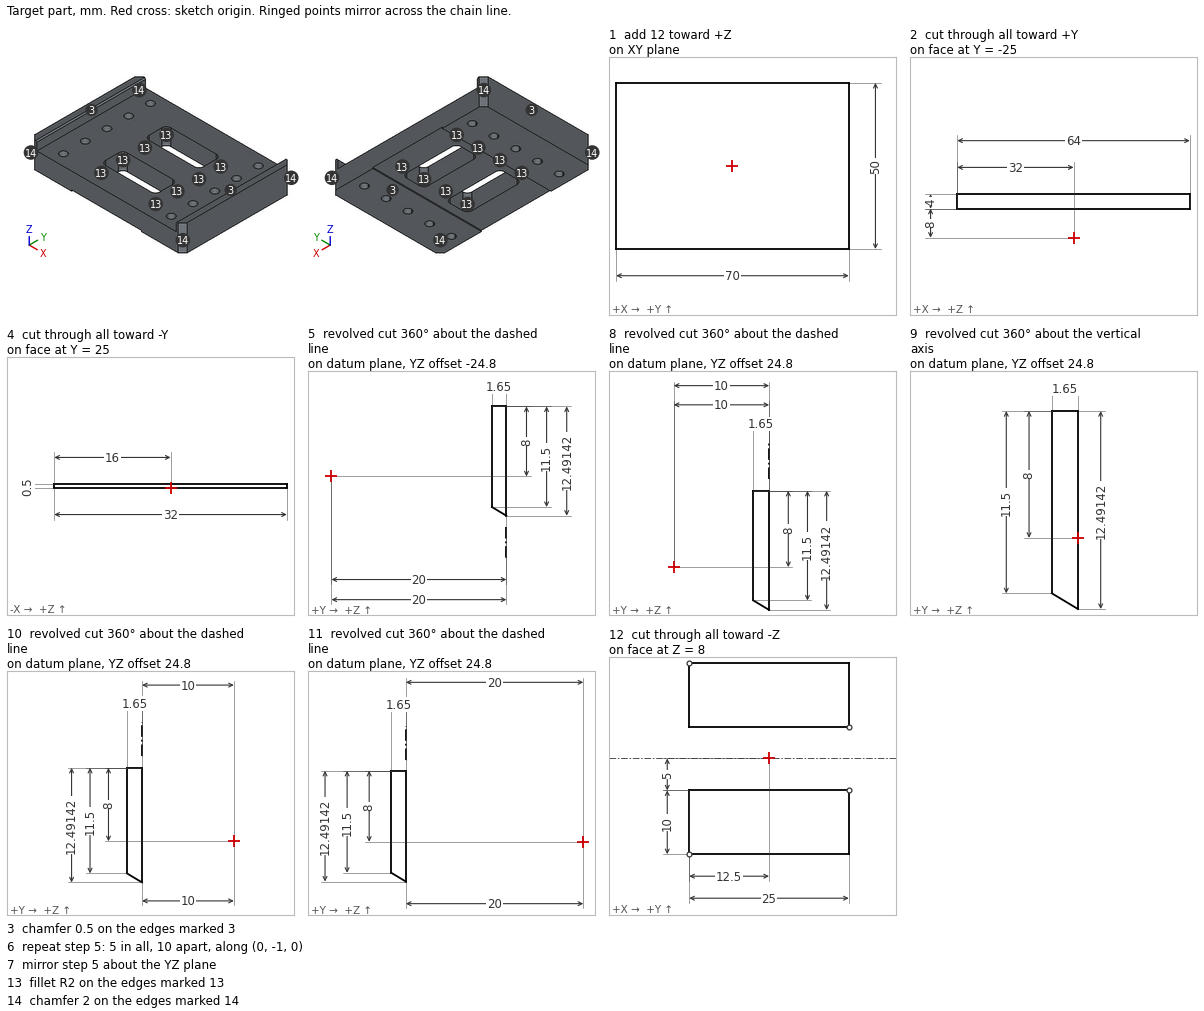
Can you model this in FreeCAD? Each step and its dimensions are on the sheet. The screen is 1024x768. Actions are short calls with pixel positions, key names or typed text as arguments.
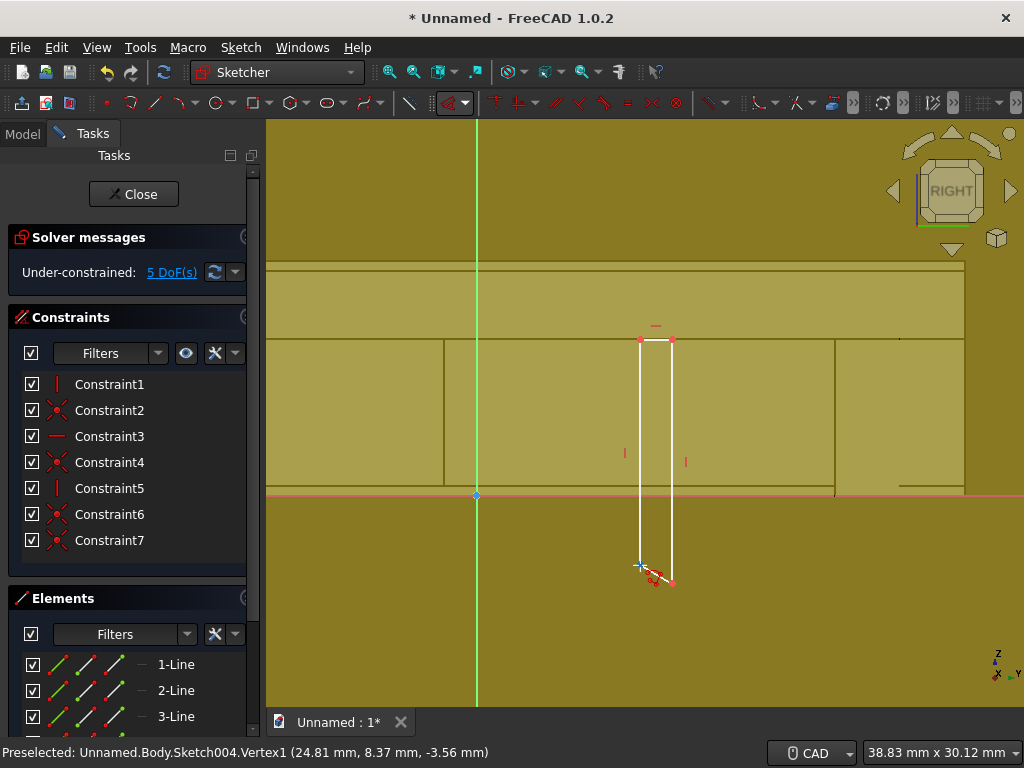
key(g)
key(l)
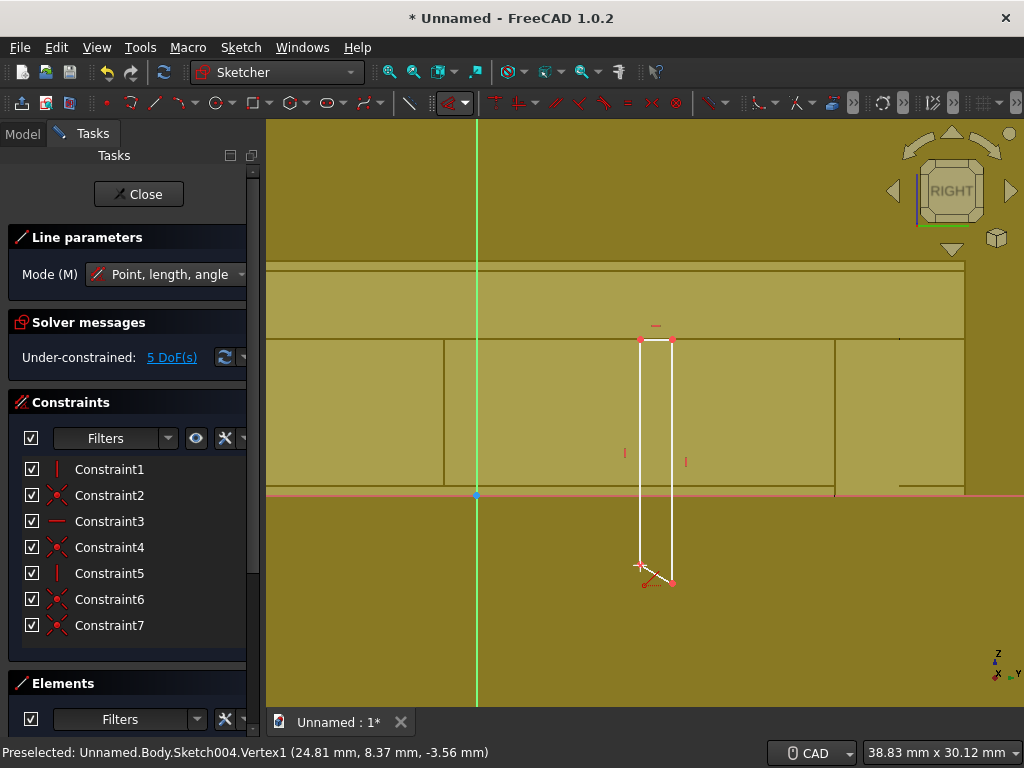
click(672, 315)
click(672, 242)
key(Escape)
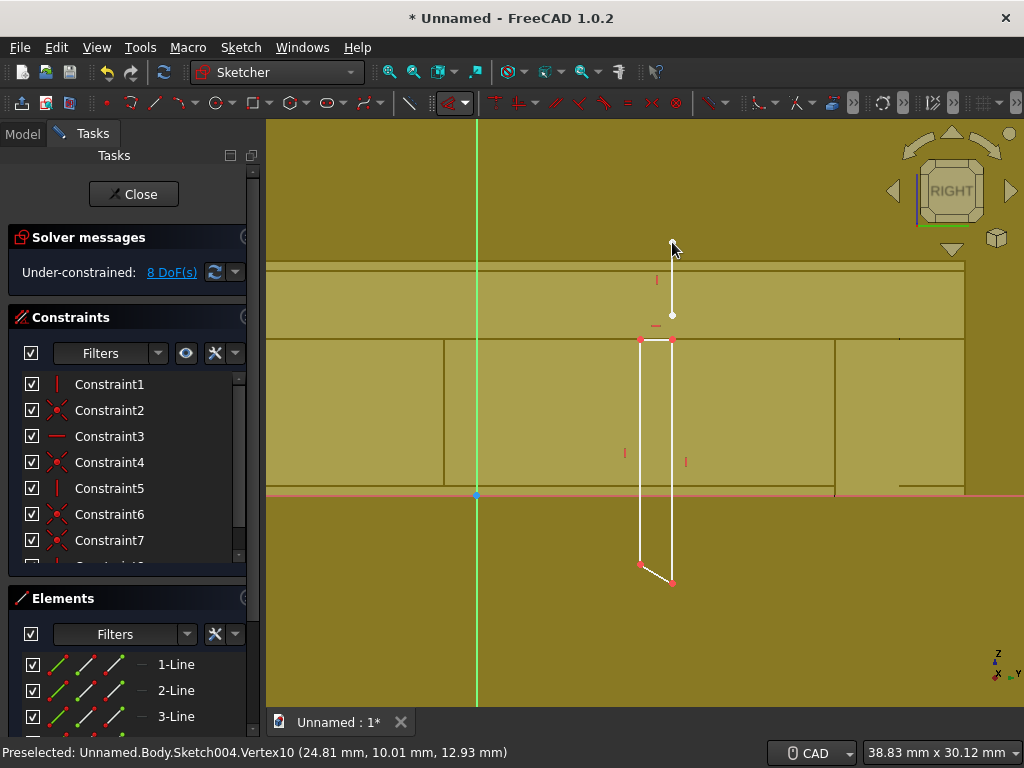
click(672, 294)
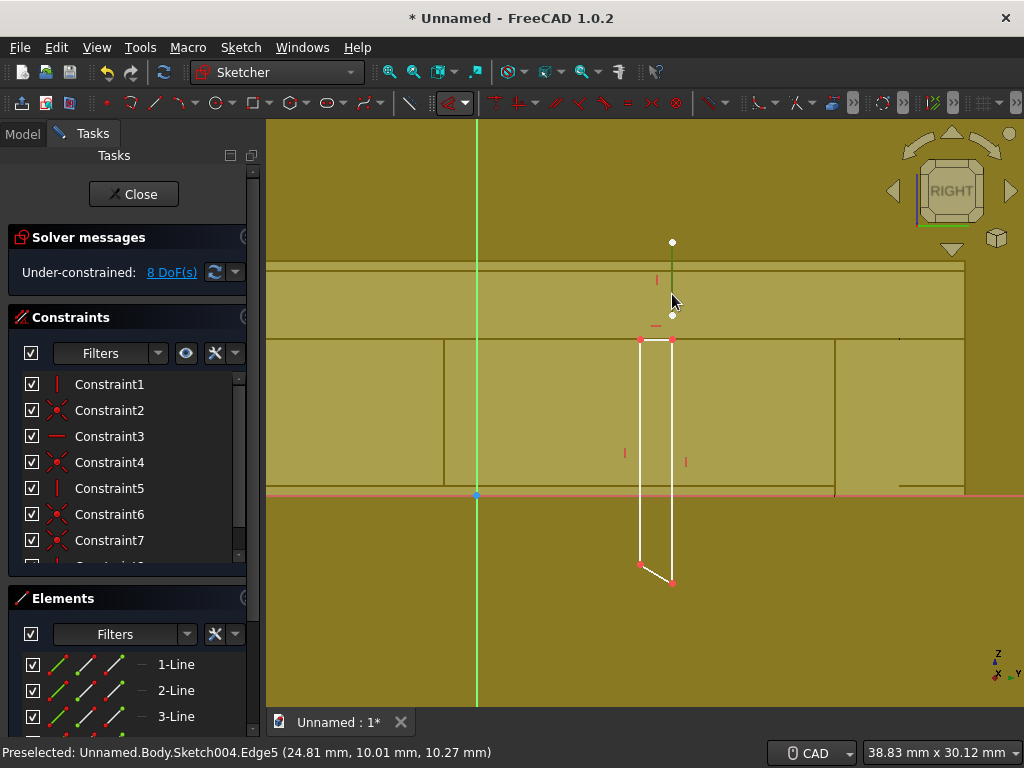
key(g)
key(n)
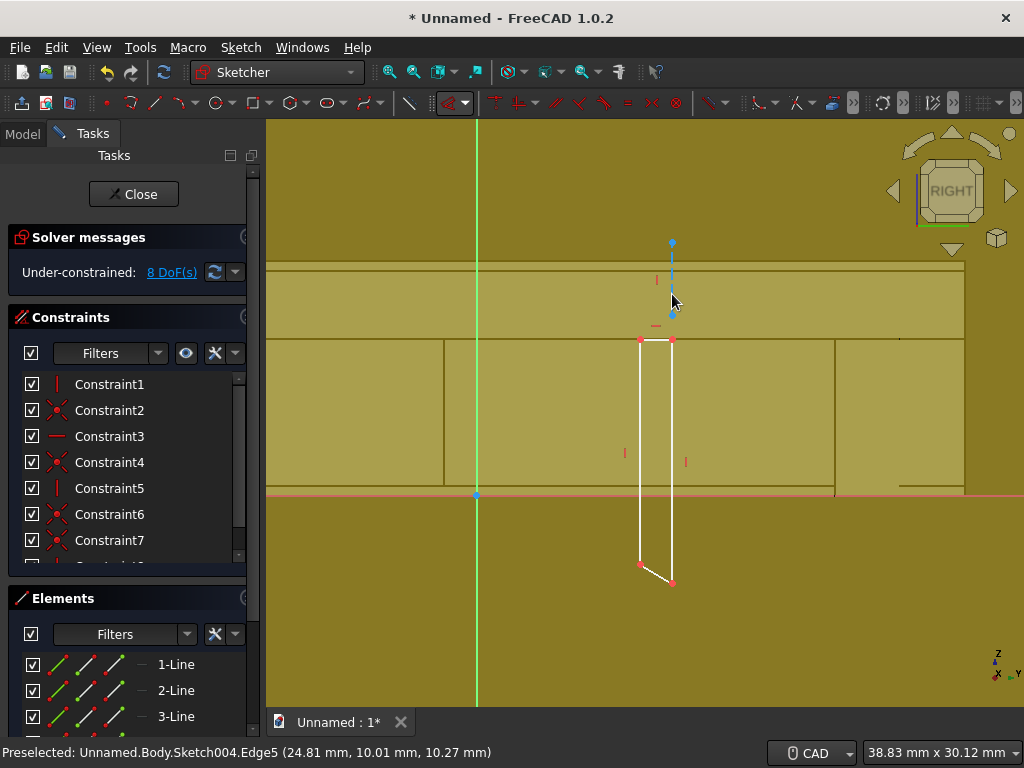
click(640, 340)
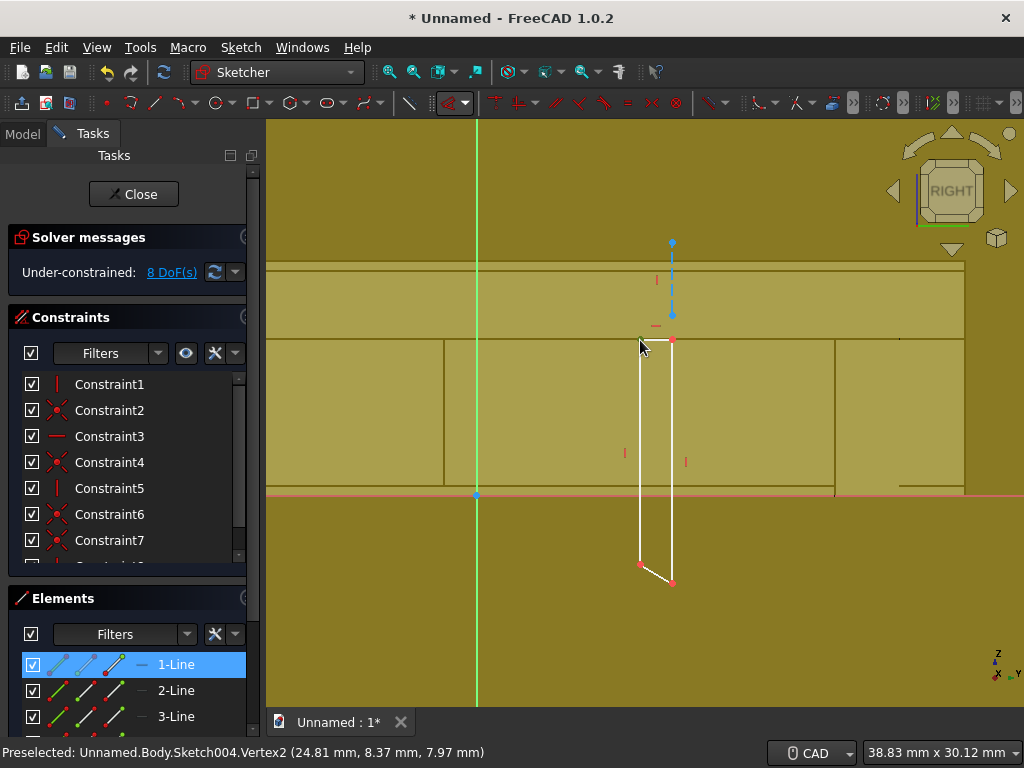
key(i)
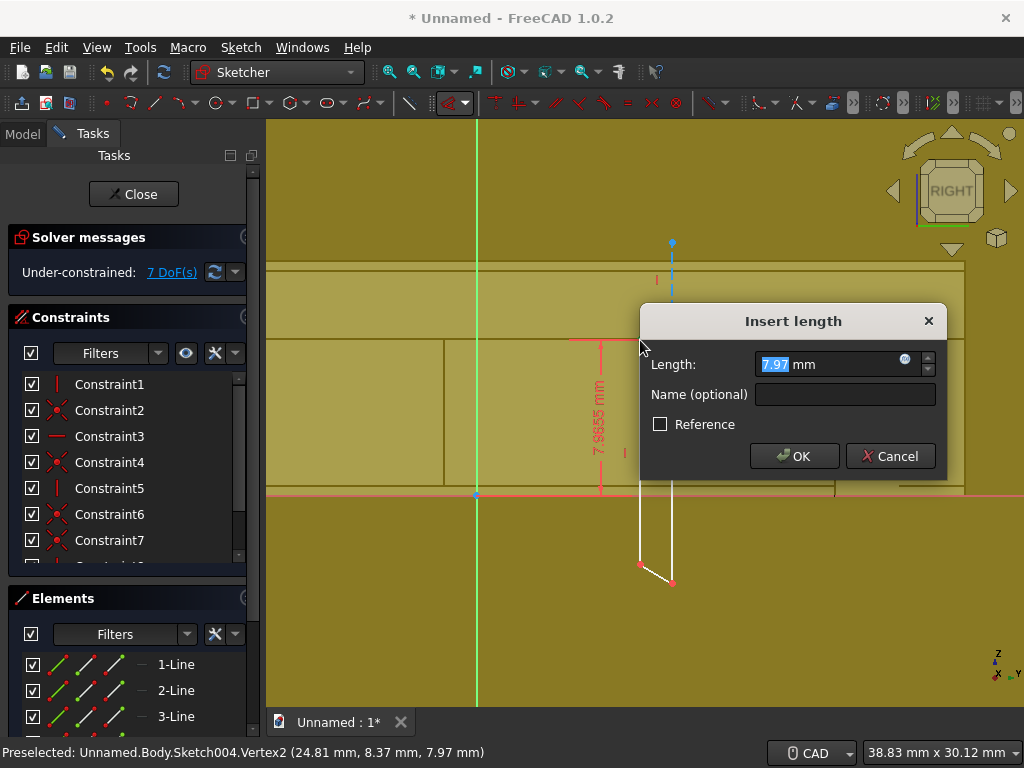
text(8)
key(Return)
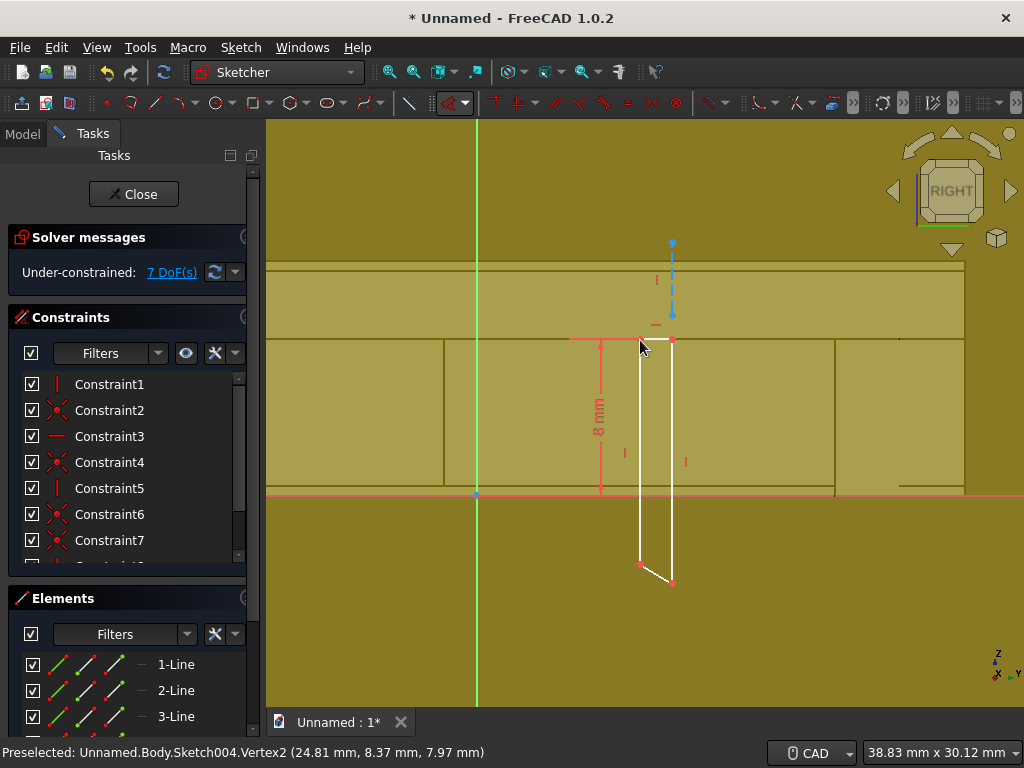
click(672, 339)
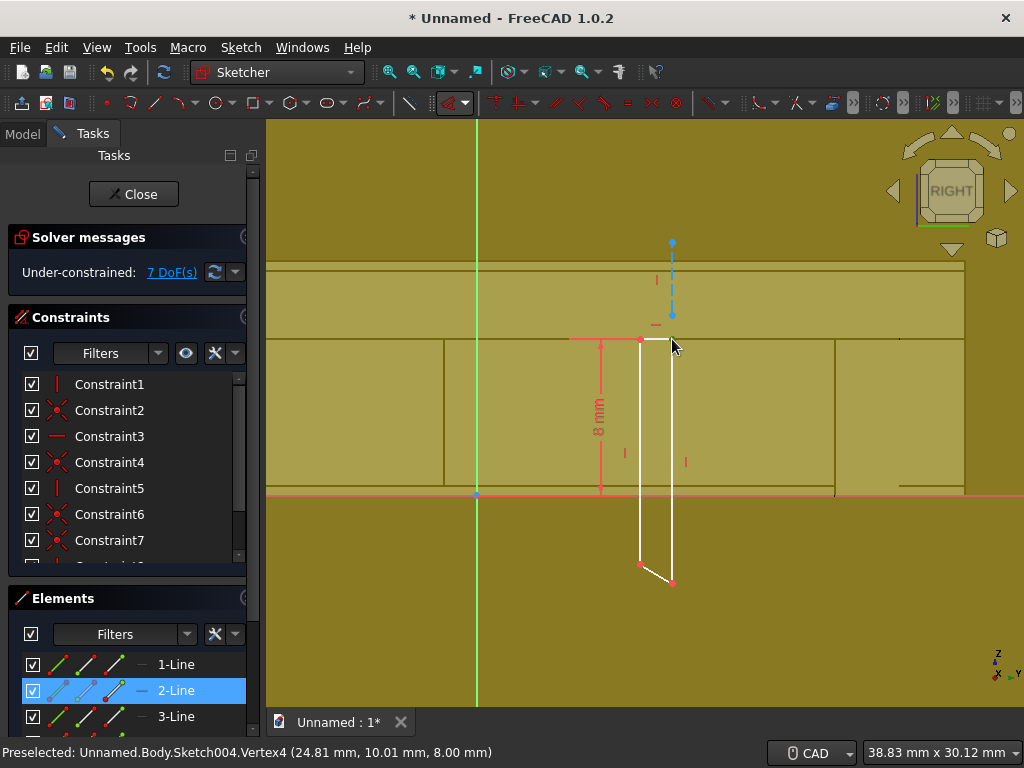
key(l)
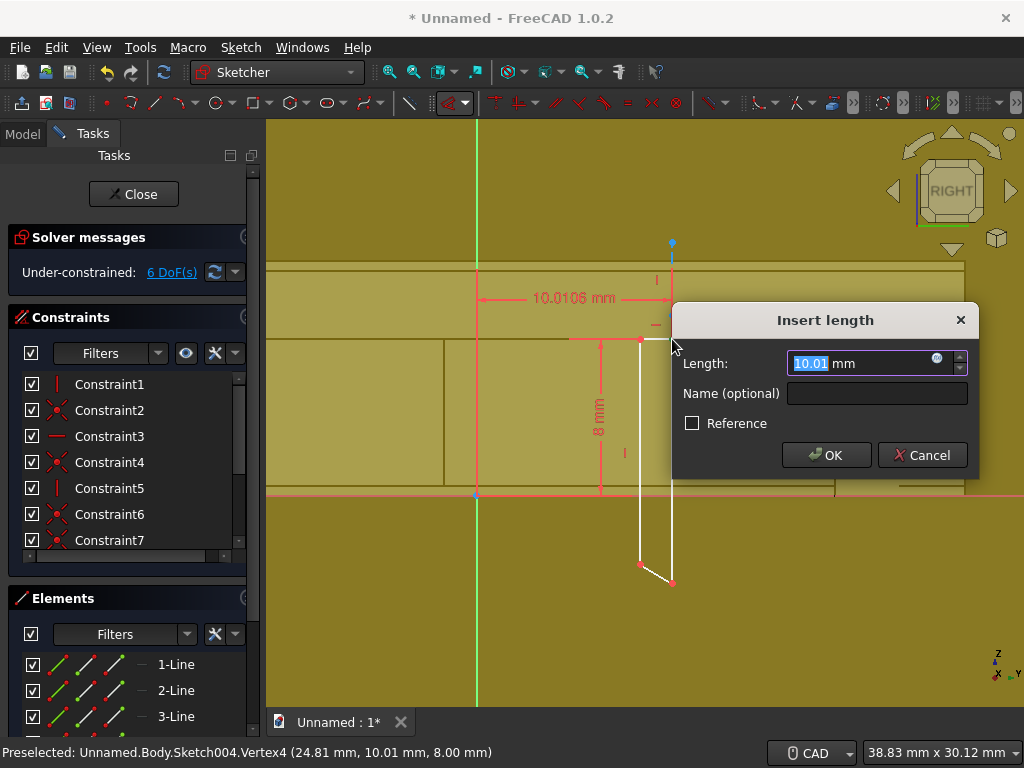
text(10)
key(Return)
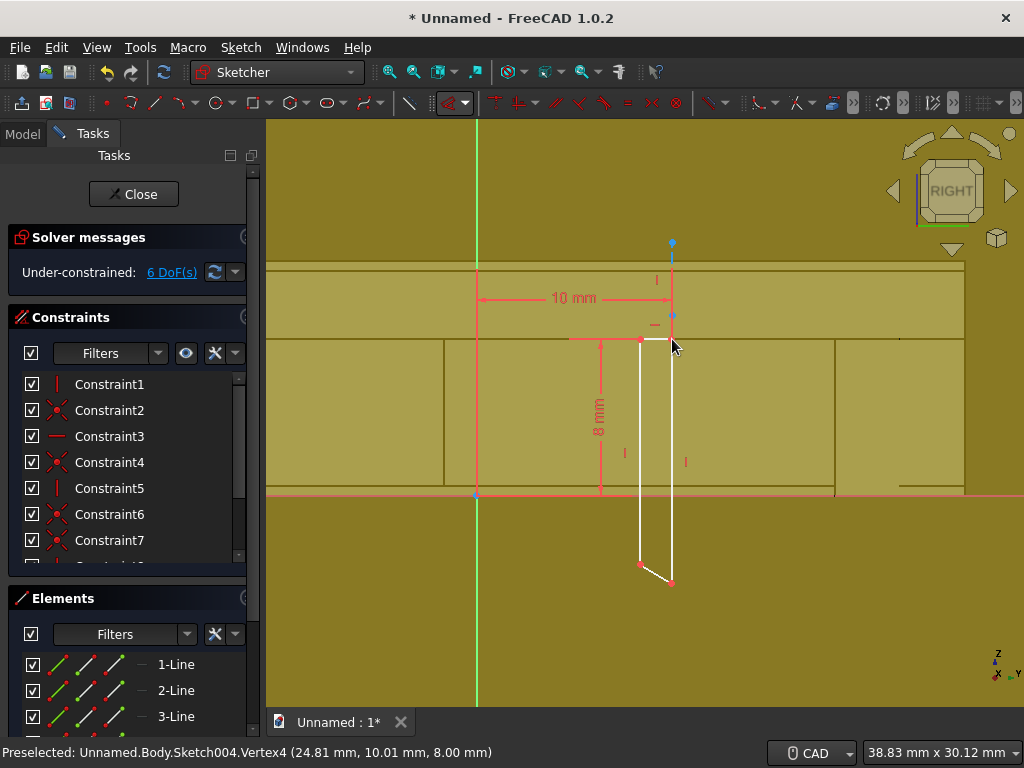
click(672, 316)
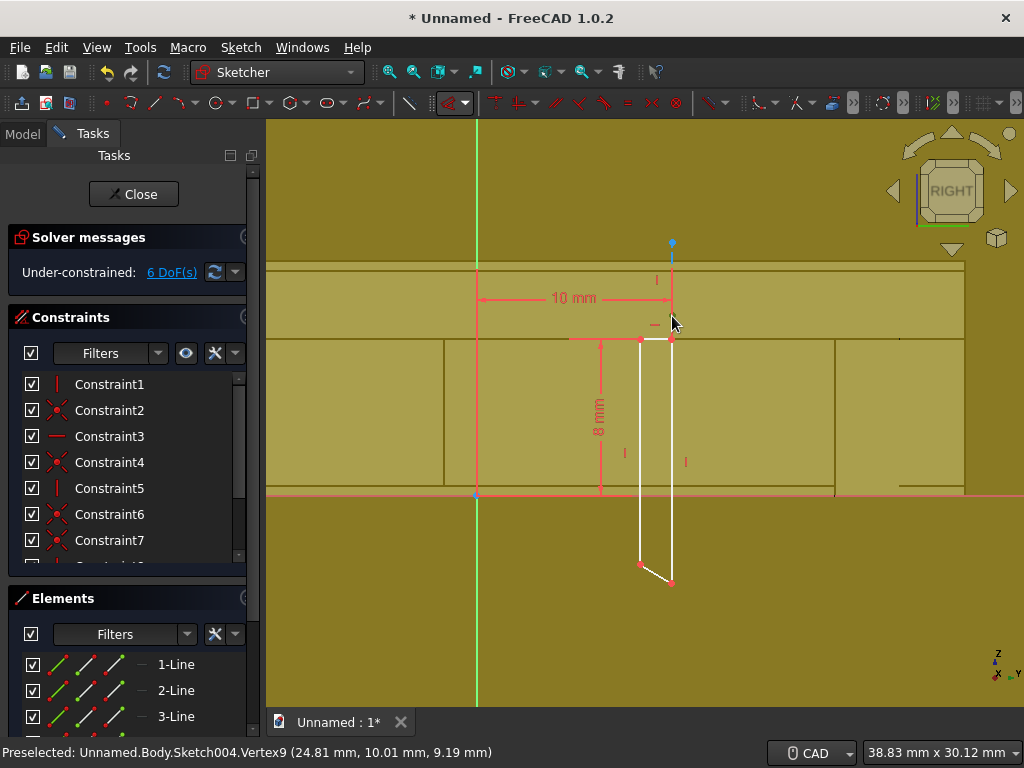
key(l)